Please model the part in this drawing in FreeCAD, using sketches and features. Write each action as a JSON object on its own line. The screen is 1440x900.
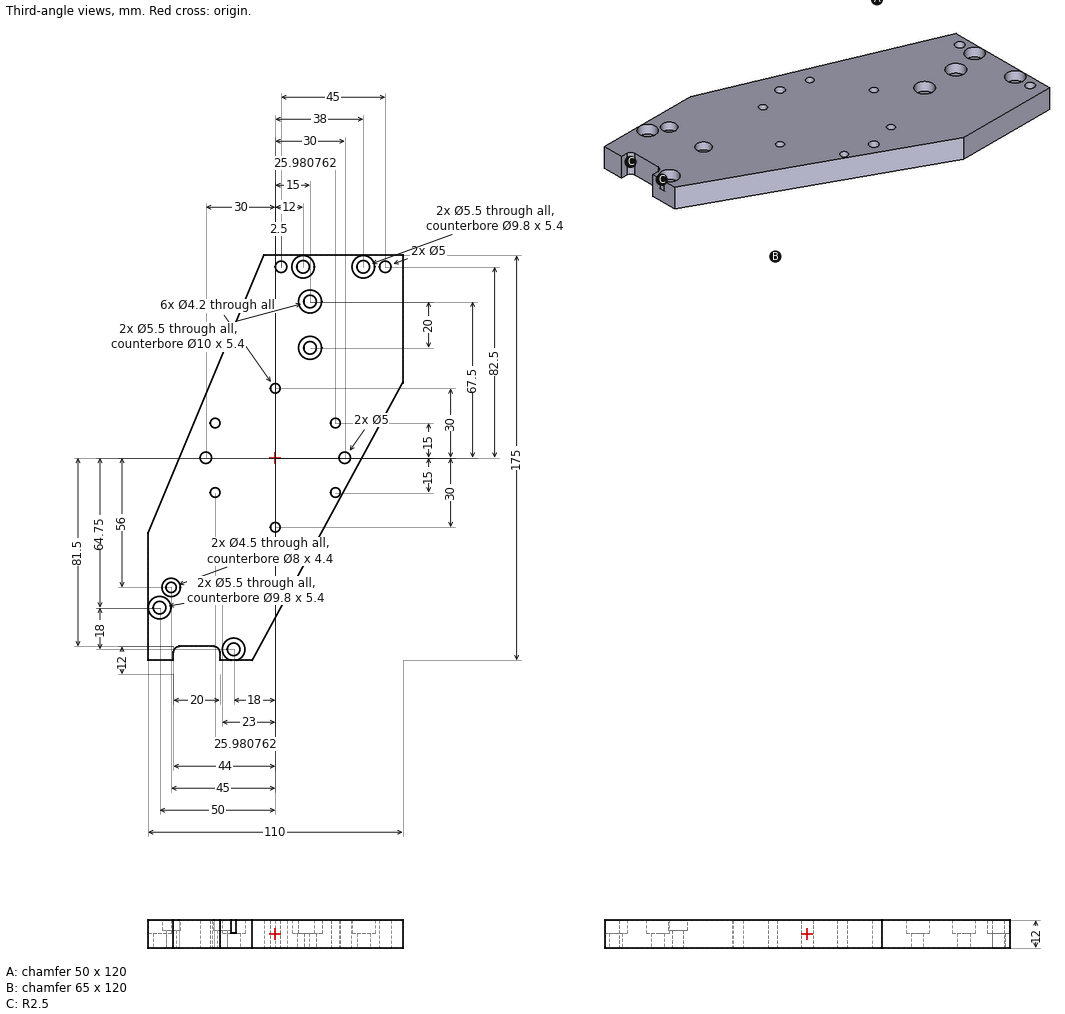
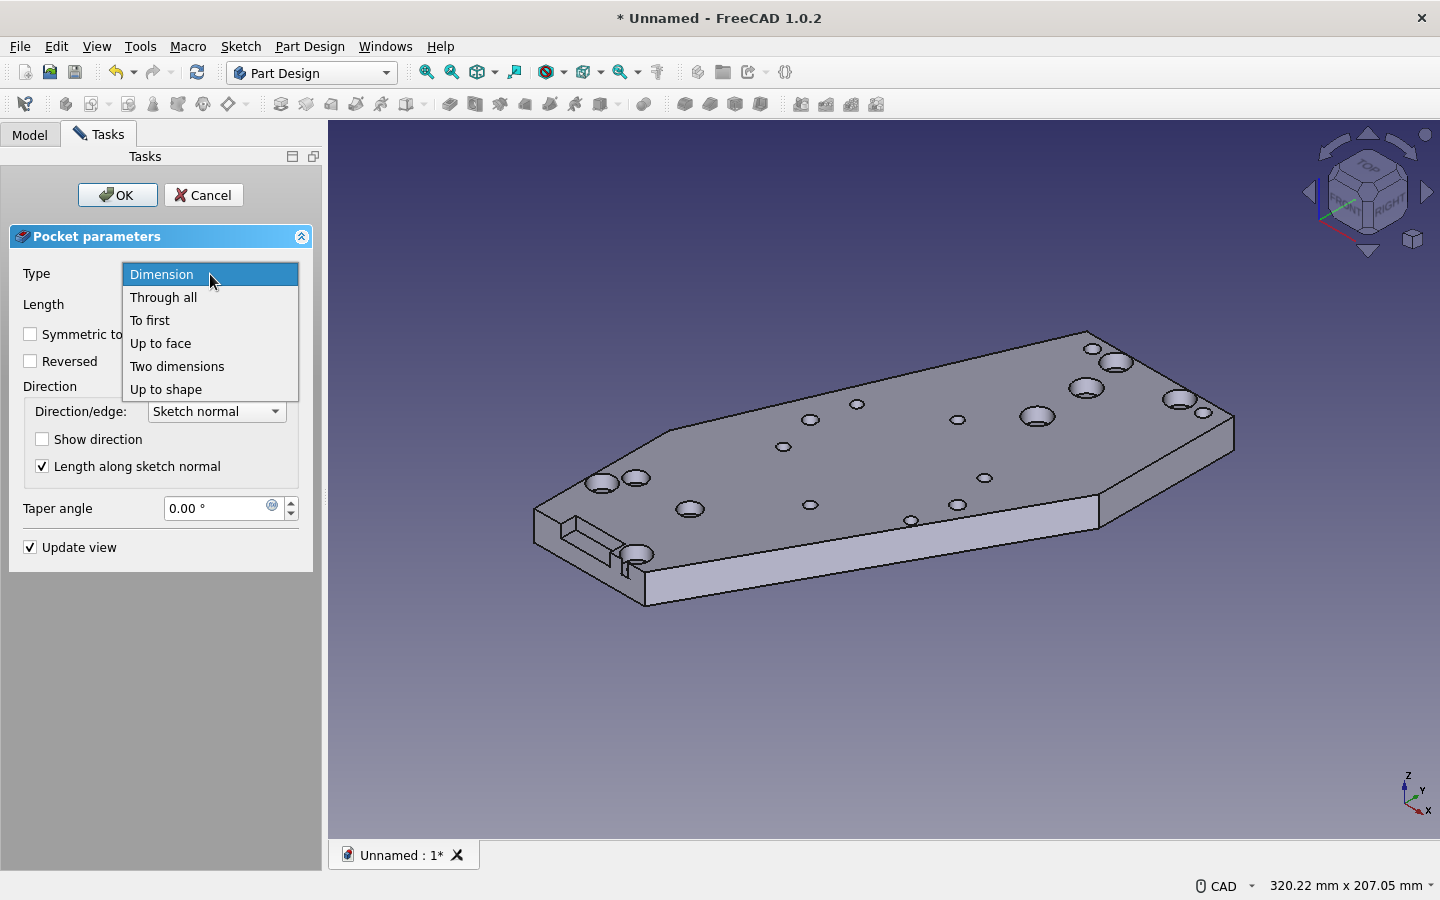
{"action": "left_click", "coordinate": [208, 298]}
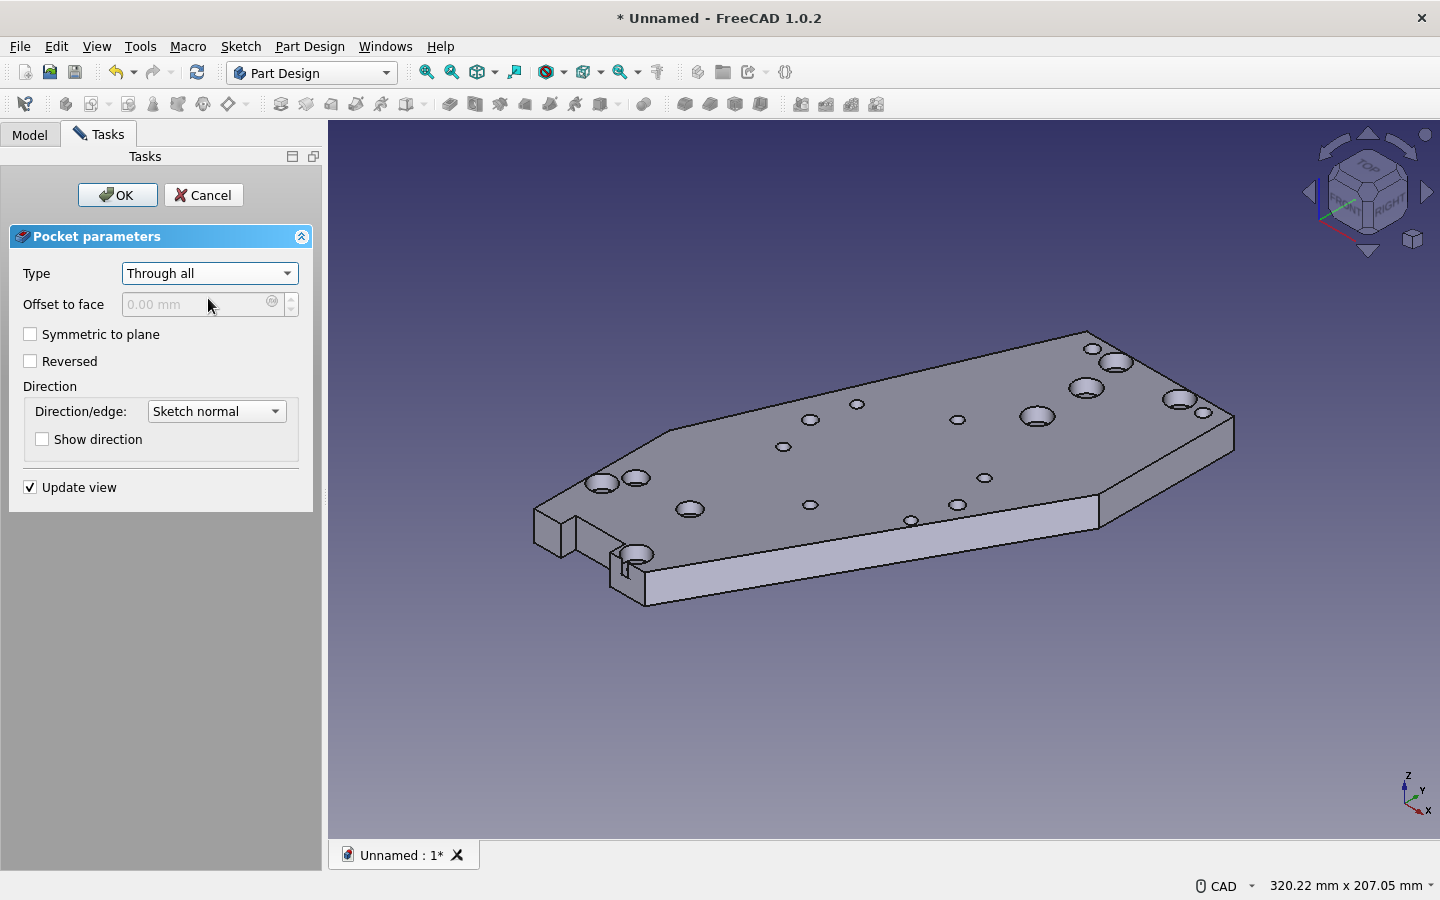
{"action": "left_click", "coordinate": [118, 195]}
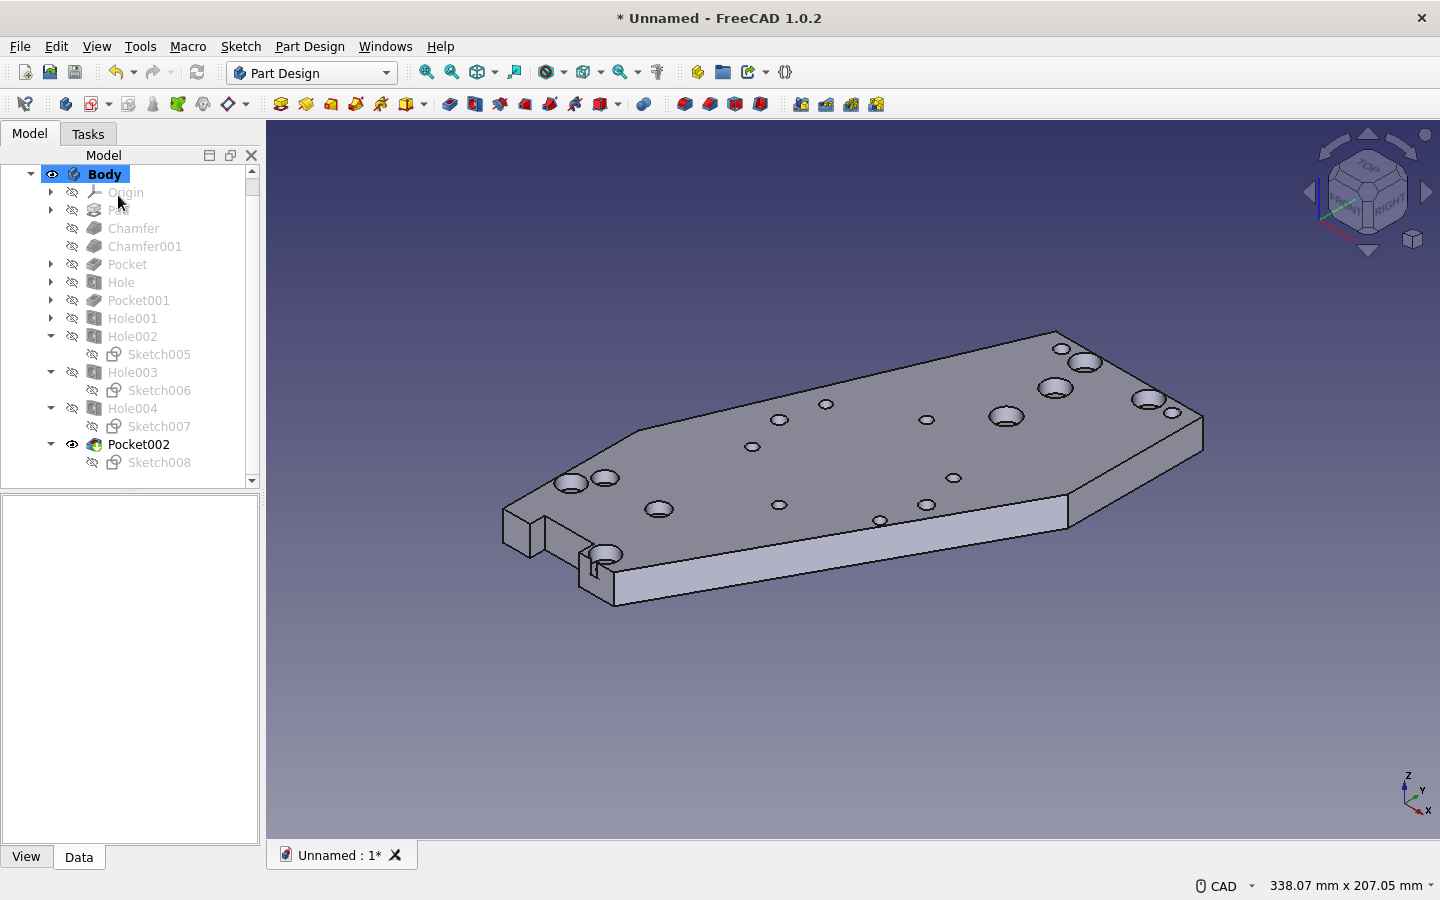
{"action": "key", "text": "2"}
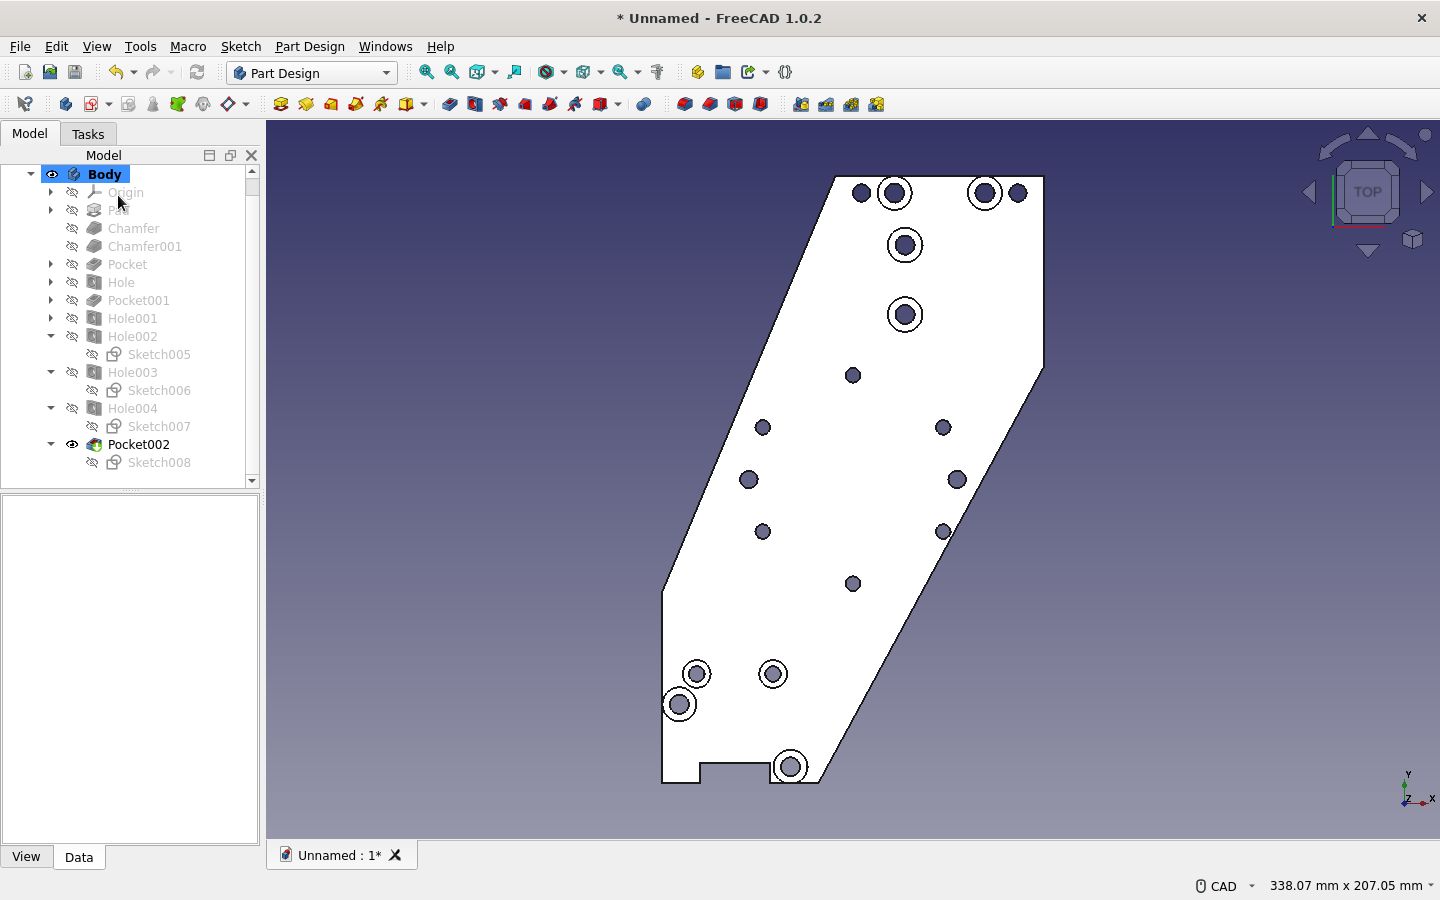
{"action": "key", "text": "0"}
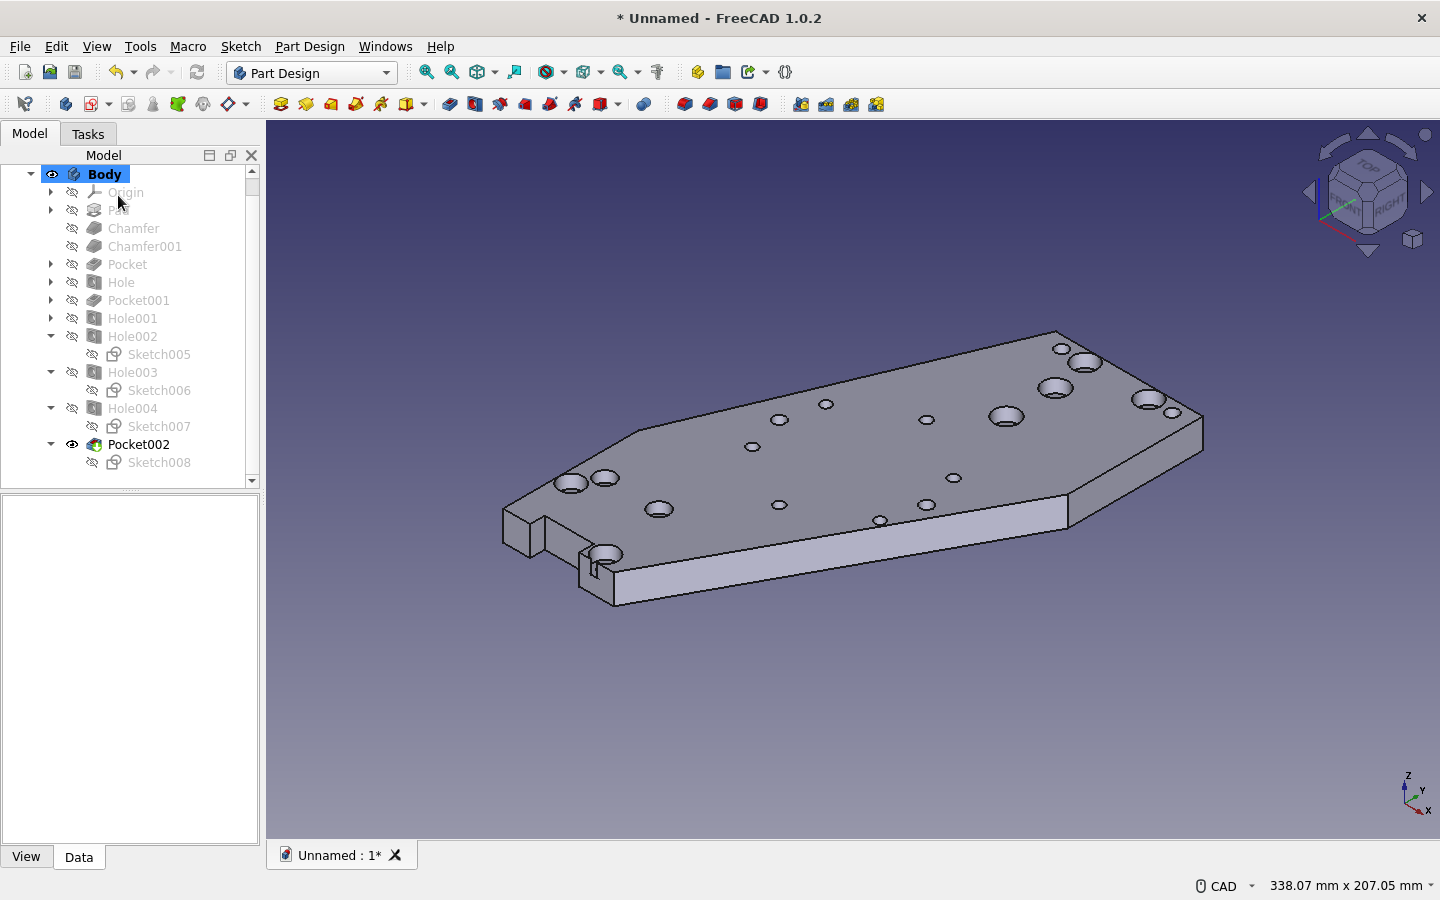
{"action": "key", "text": "1"}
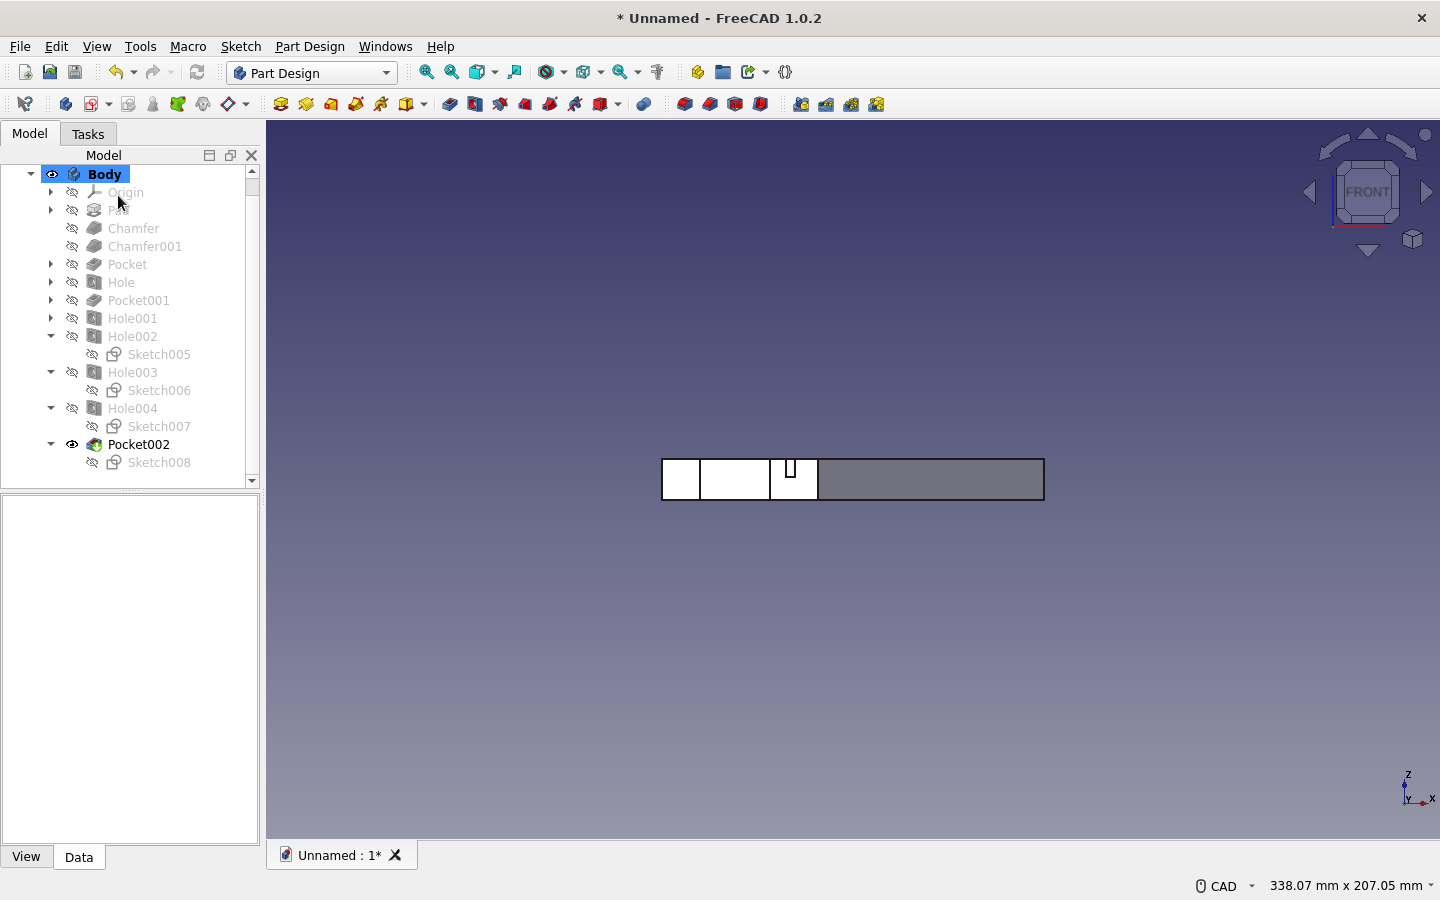
{"action": "key", "text": "v f"}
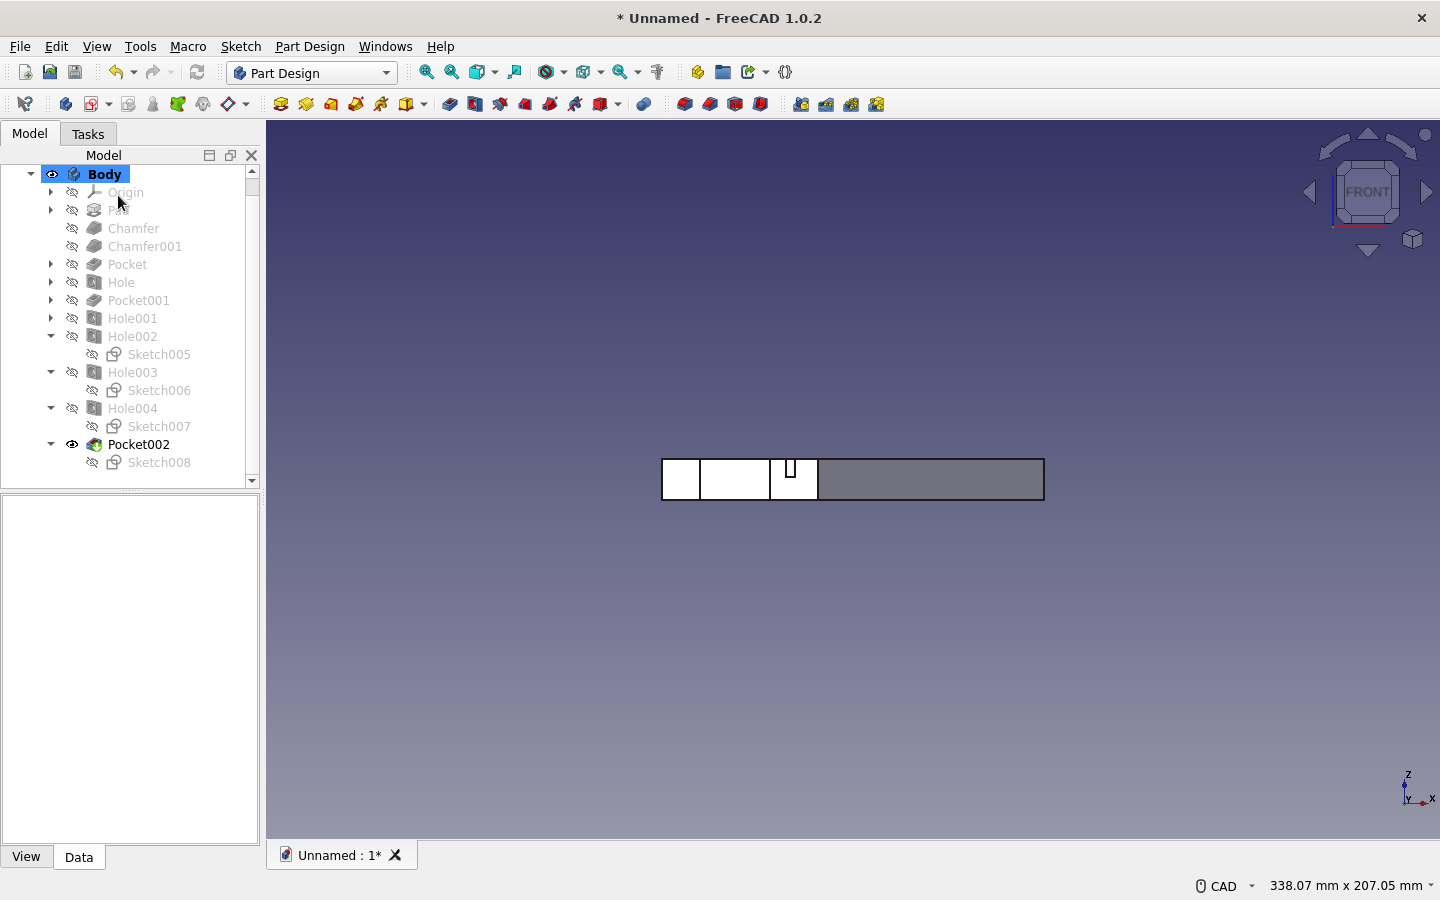
{"action": "key", "text": "3"}